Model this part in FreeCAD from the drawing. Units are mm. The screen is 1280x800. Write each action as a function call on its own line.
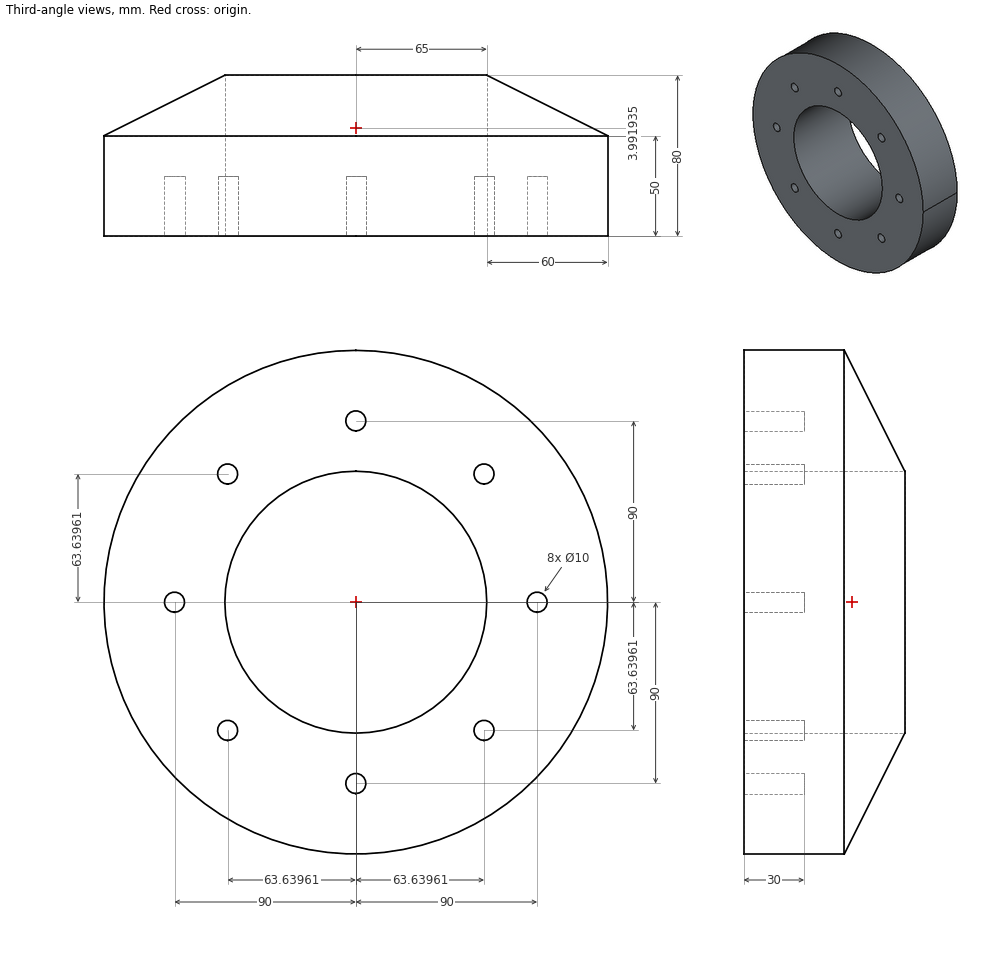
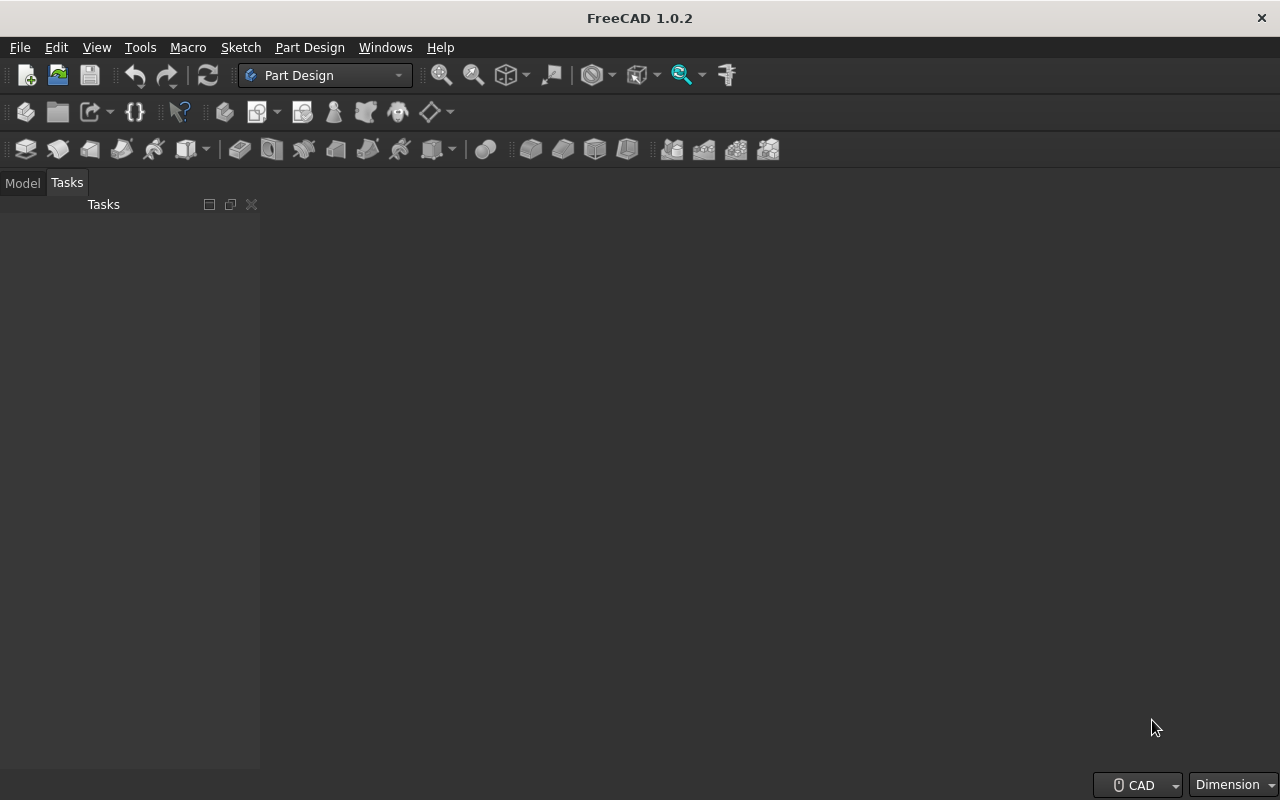
key(ctrl+n)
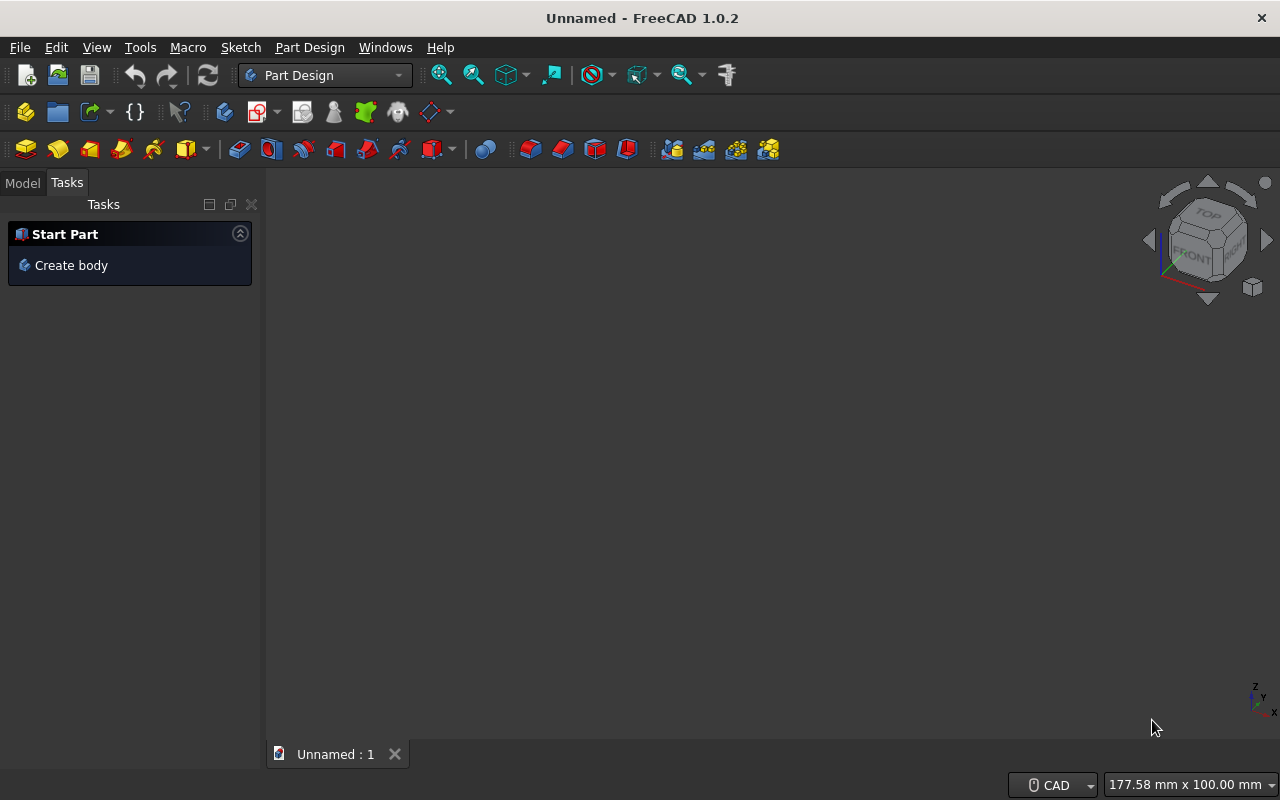
click(258, 112)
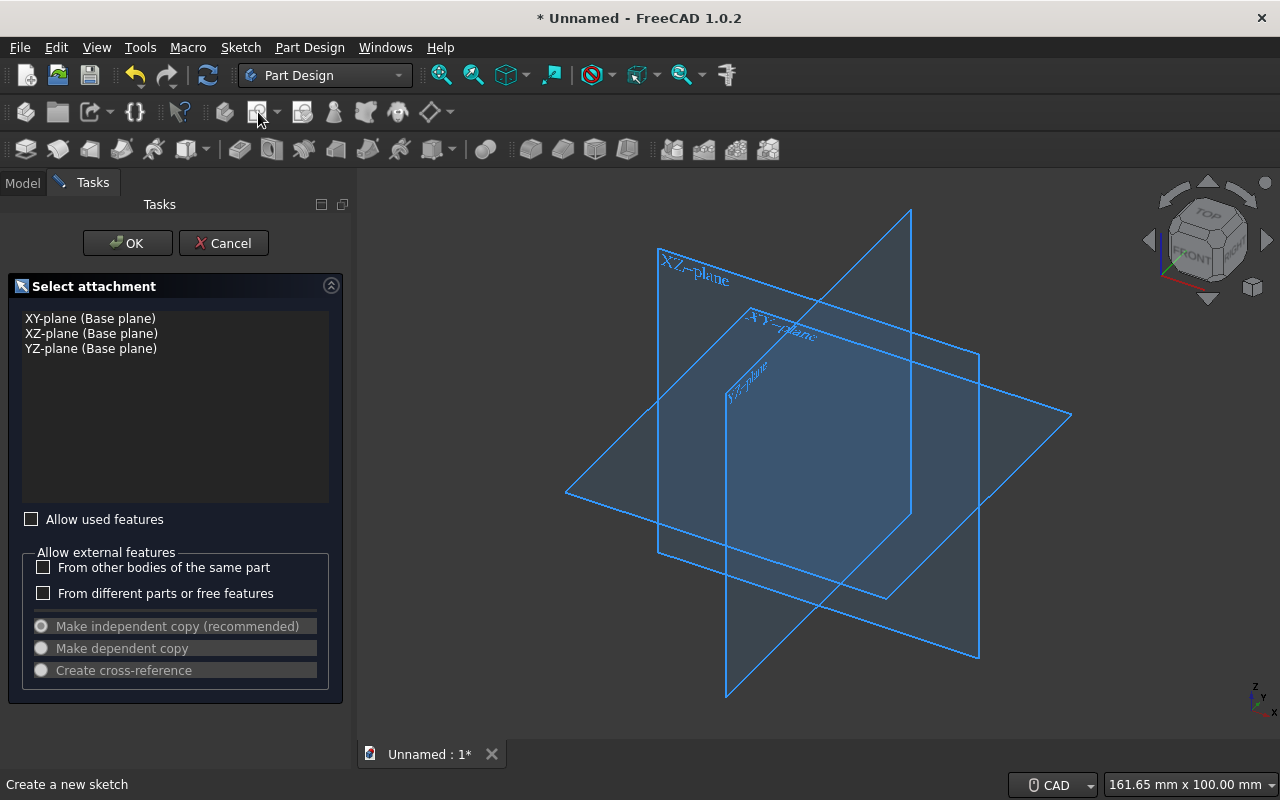
click(82, 318)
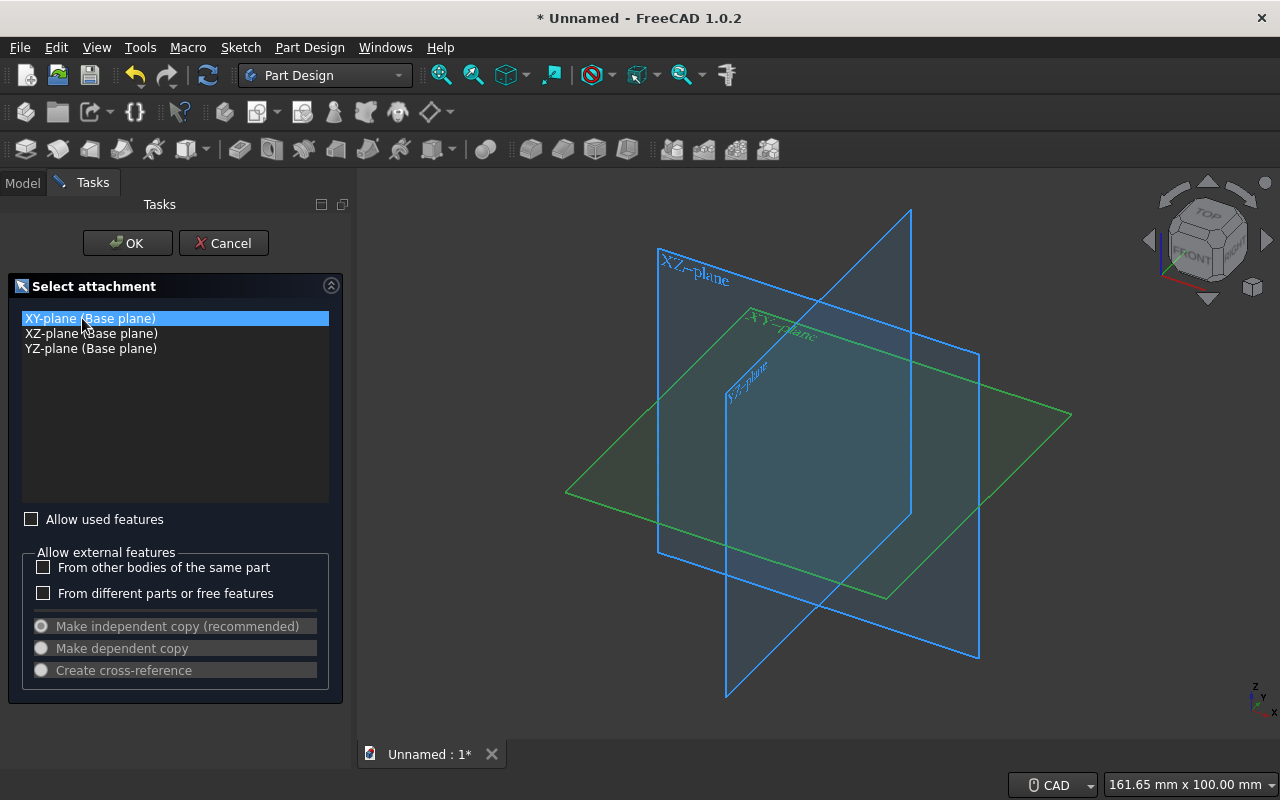
click(128, 243)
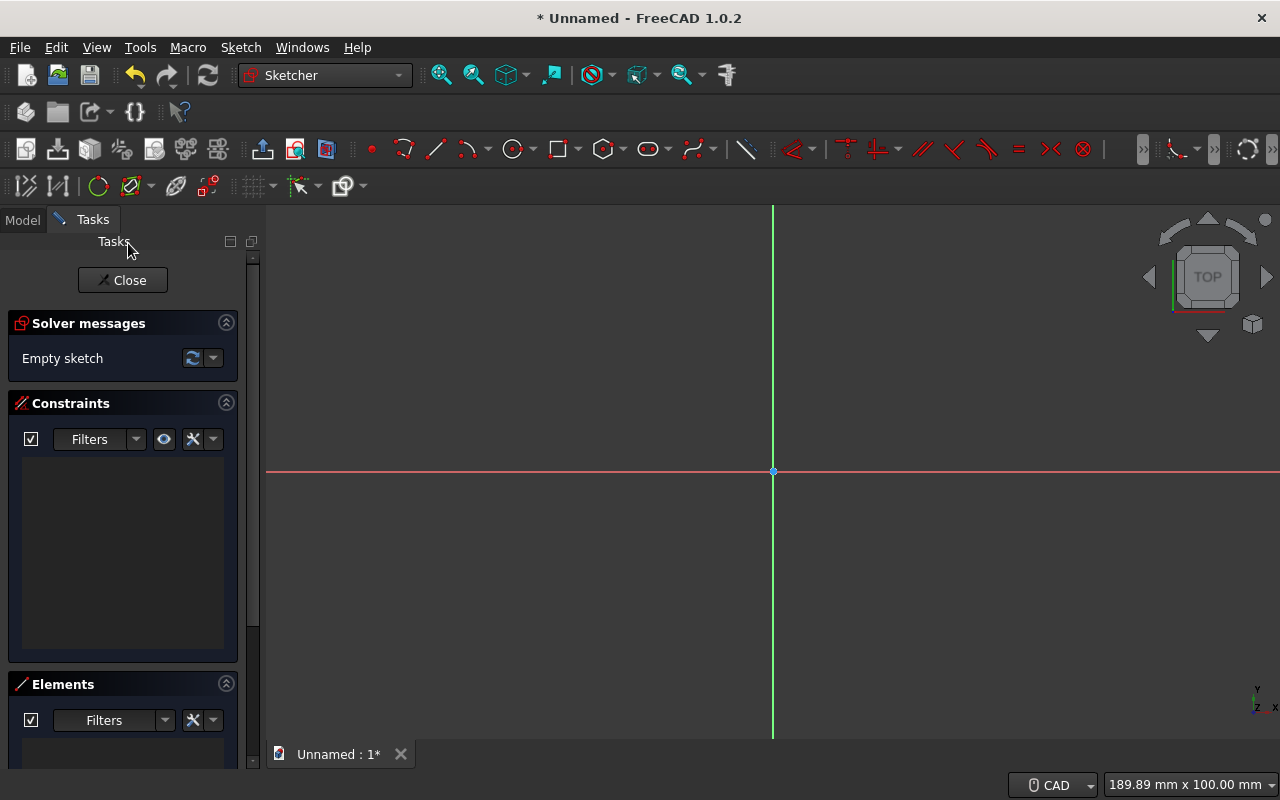
scroll(294, 320, down, 2)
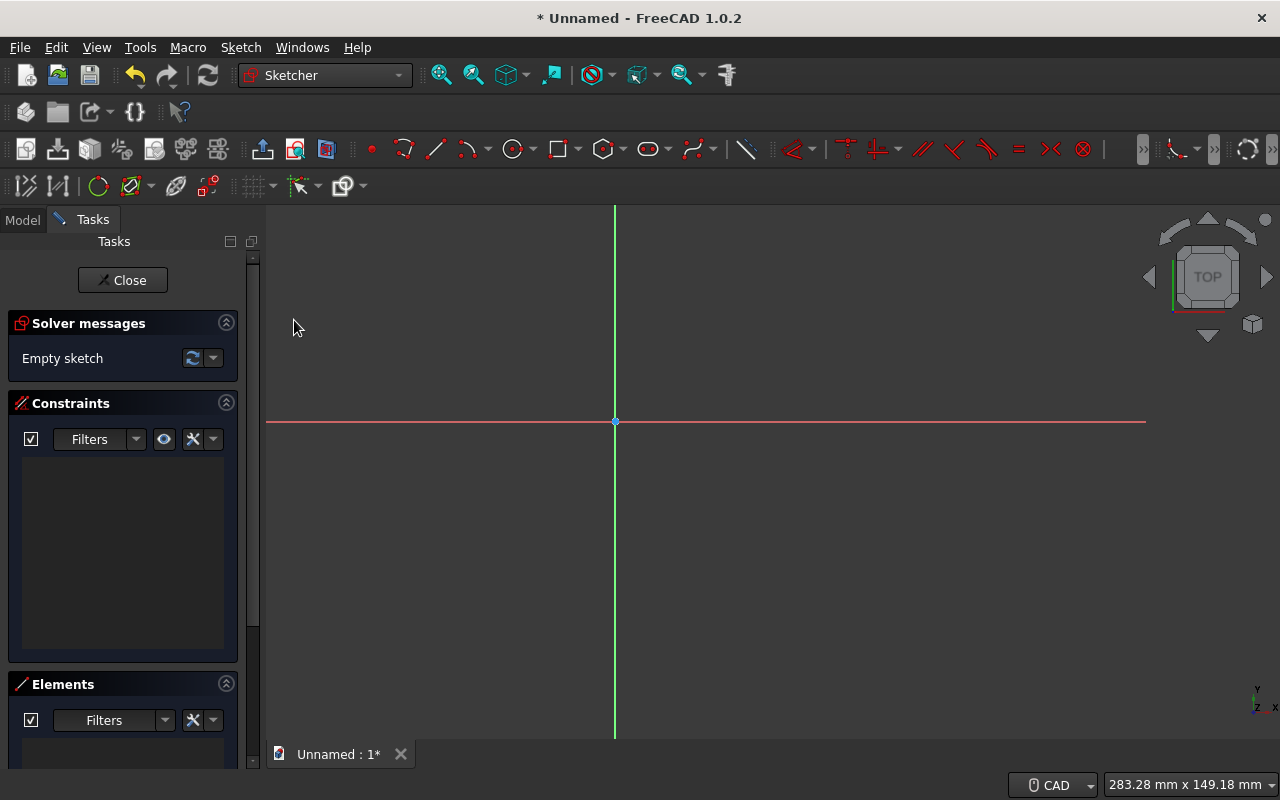
click(404, 150)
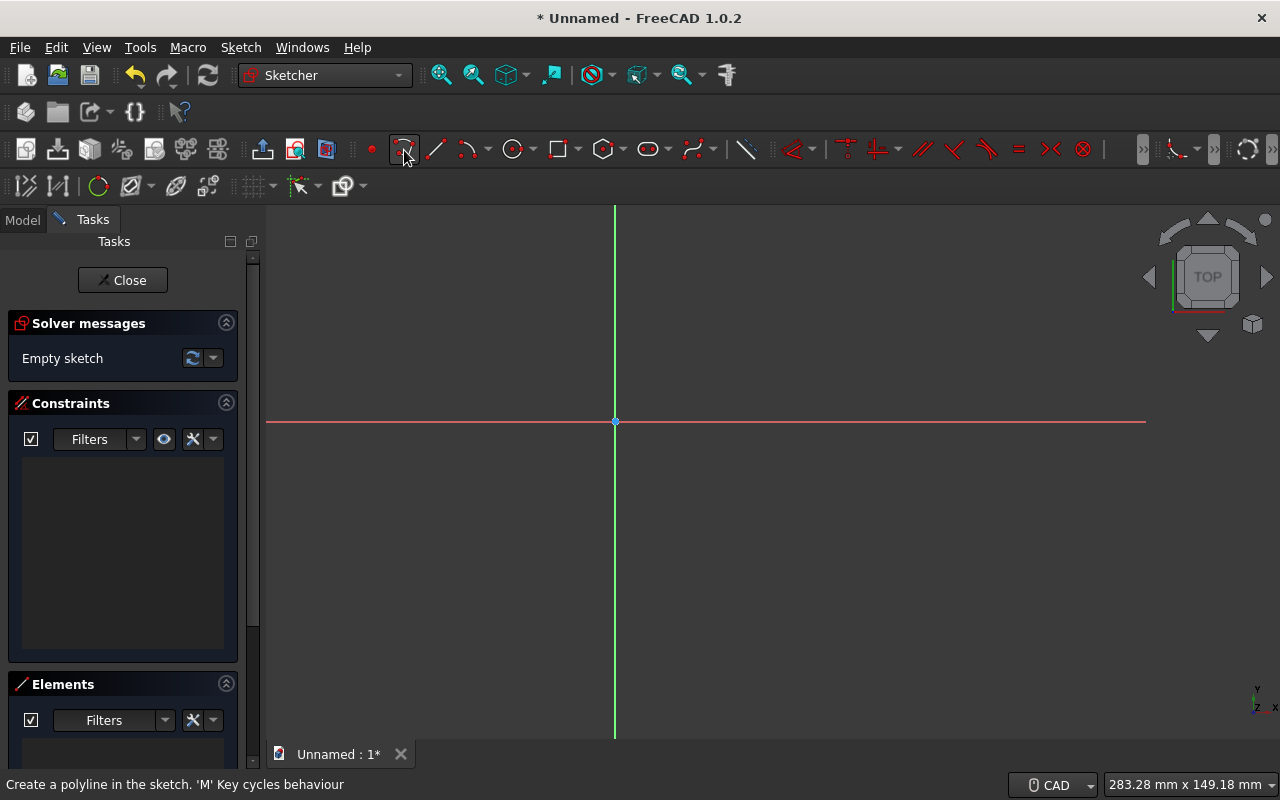
click(848, 329)
click(848, 615)
click(1063, 615)
click(1063, 436)
click(848, 330)
key(Escape)
key(Escape)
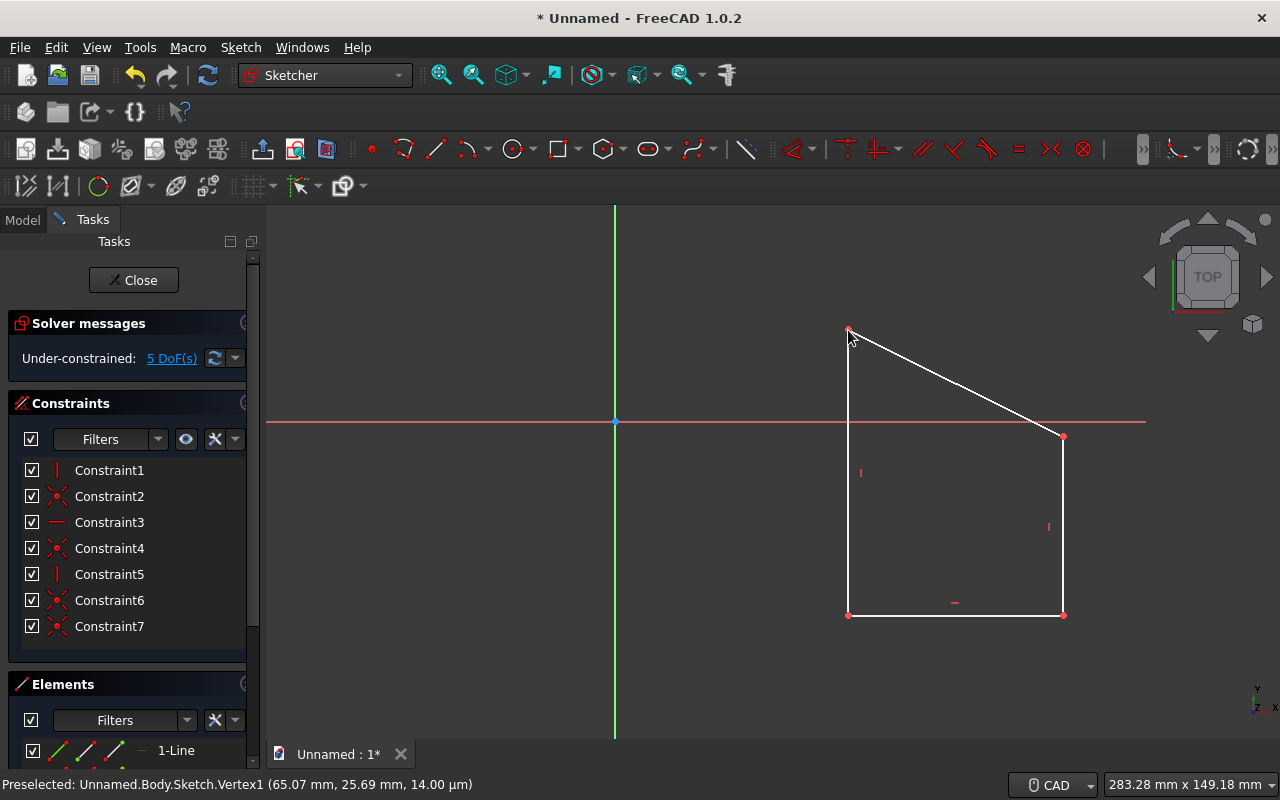
click(792, 150)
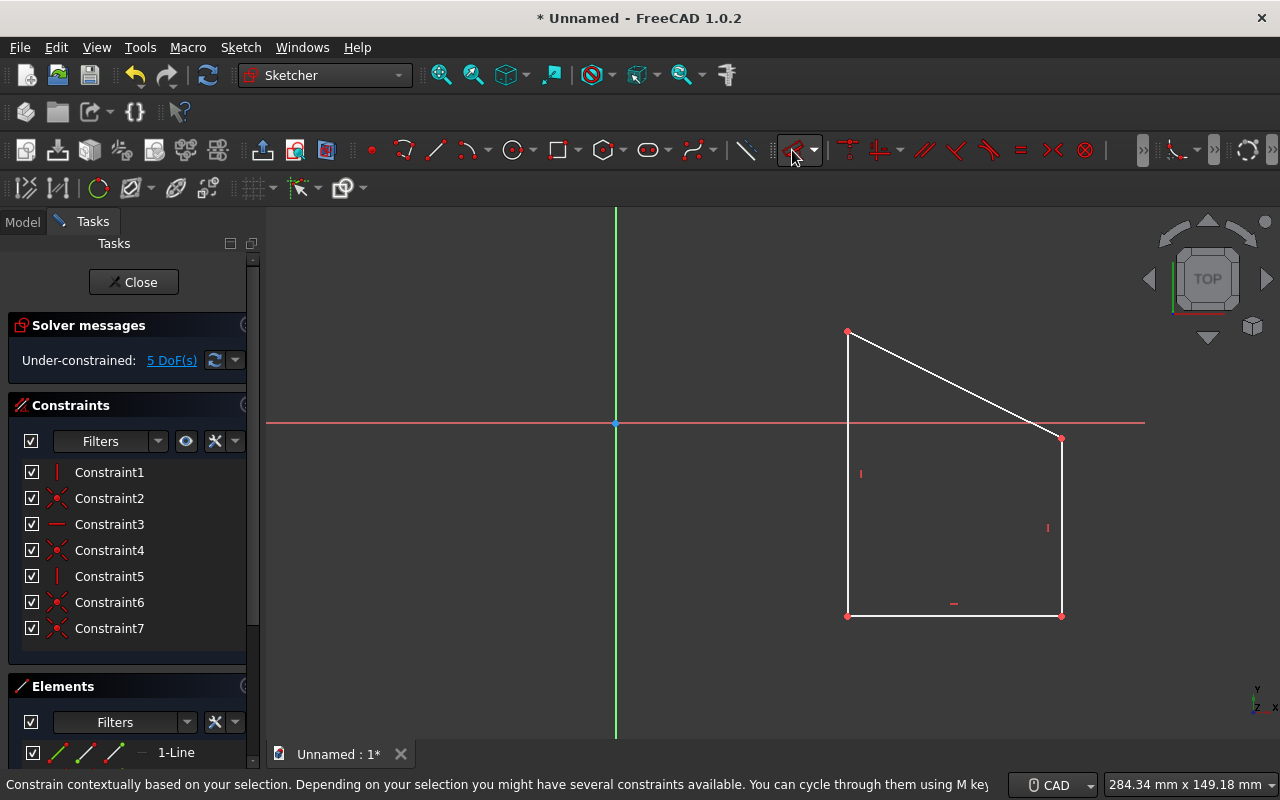
click(848, 531)
click(882, 474)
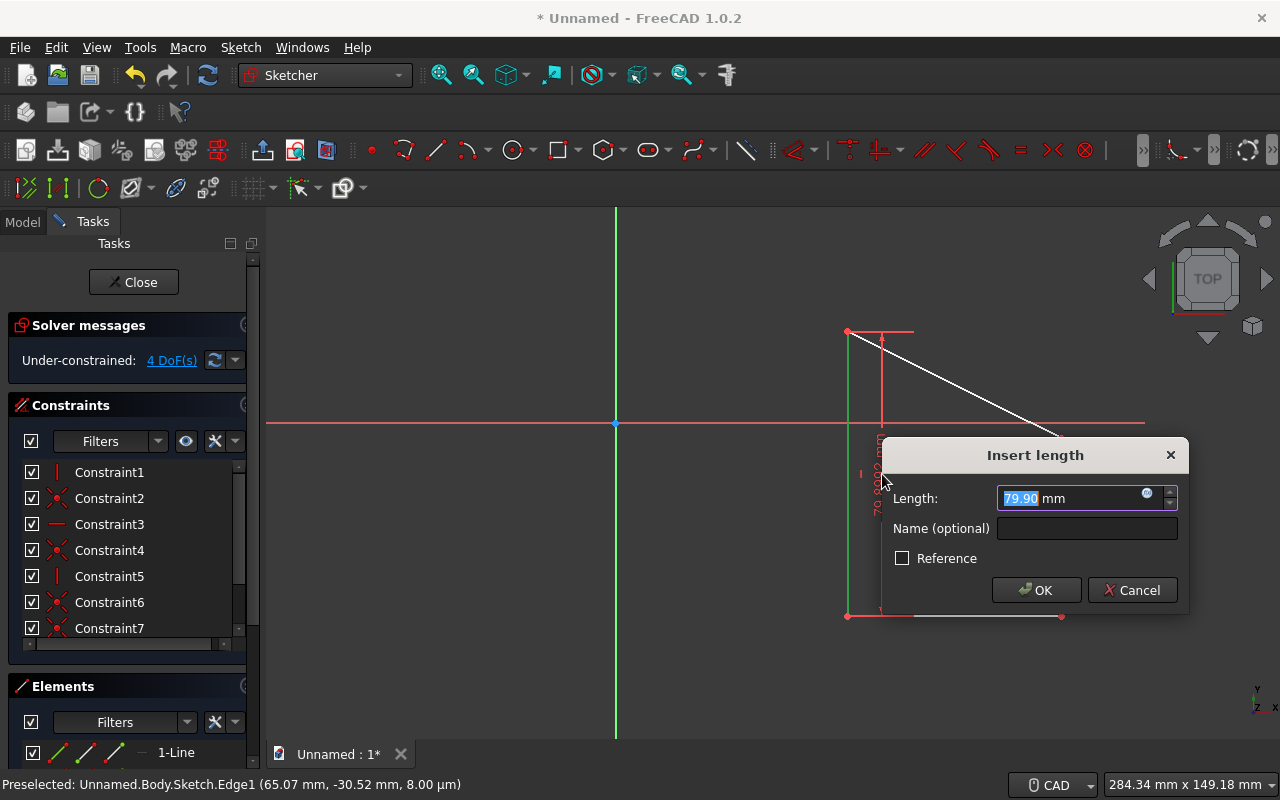
text(80)
key(Return)